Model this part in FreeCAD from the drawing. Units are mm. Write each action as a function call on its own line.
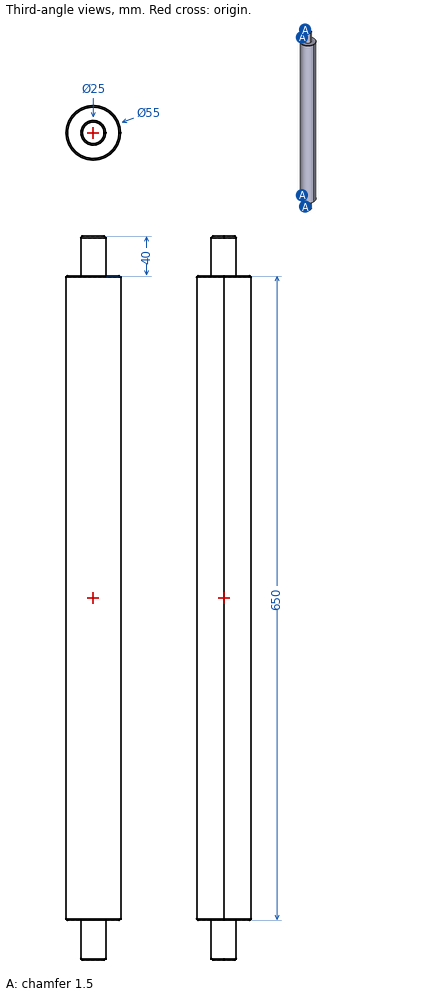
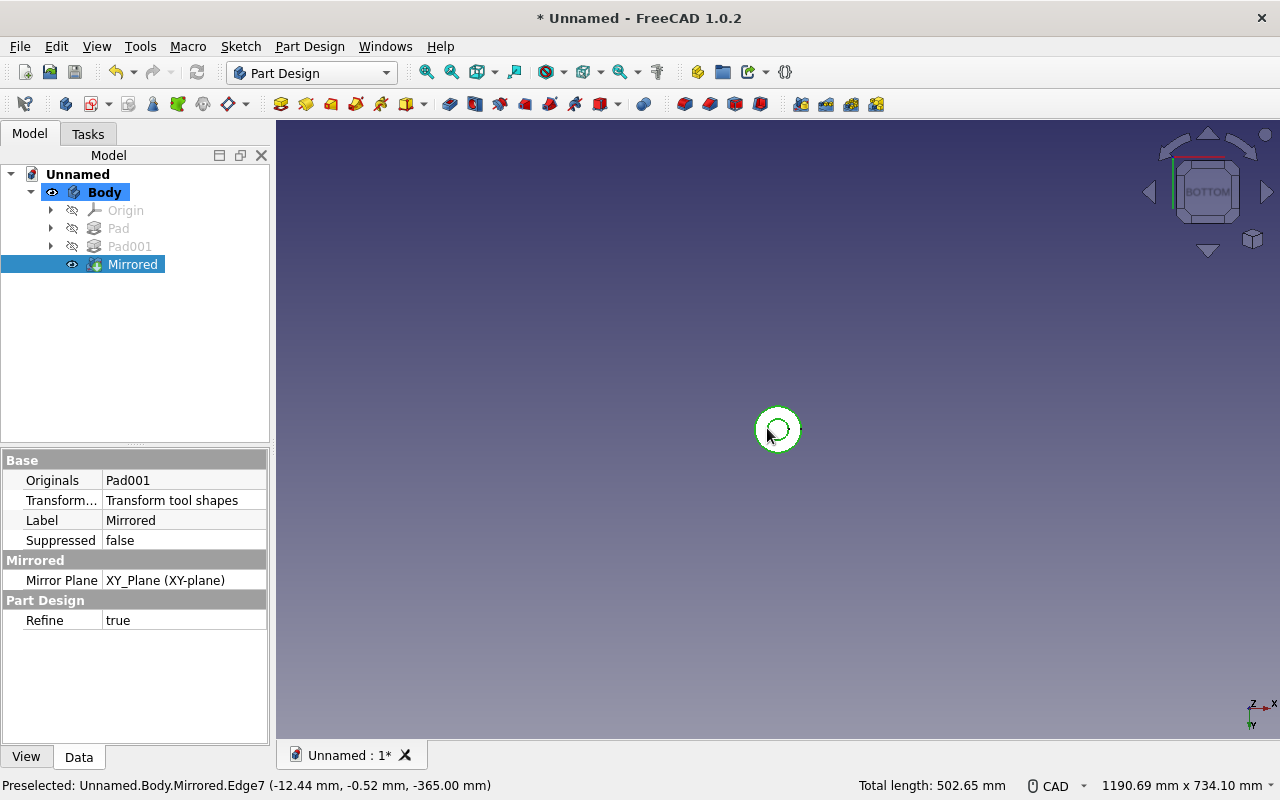
click(710, 104)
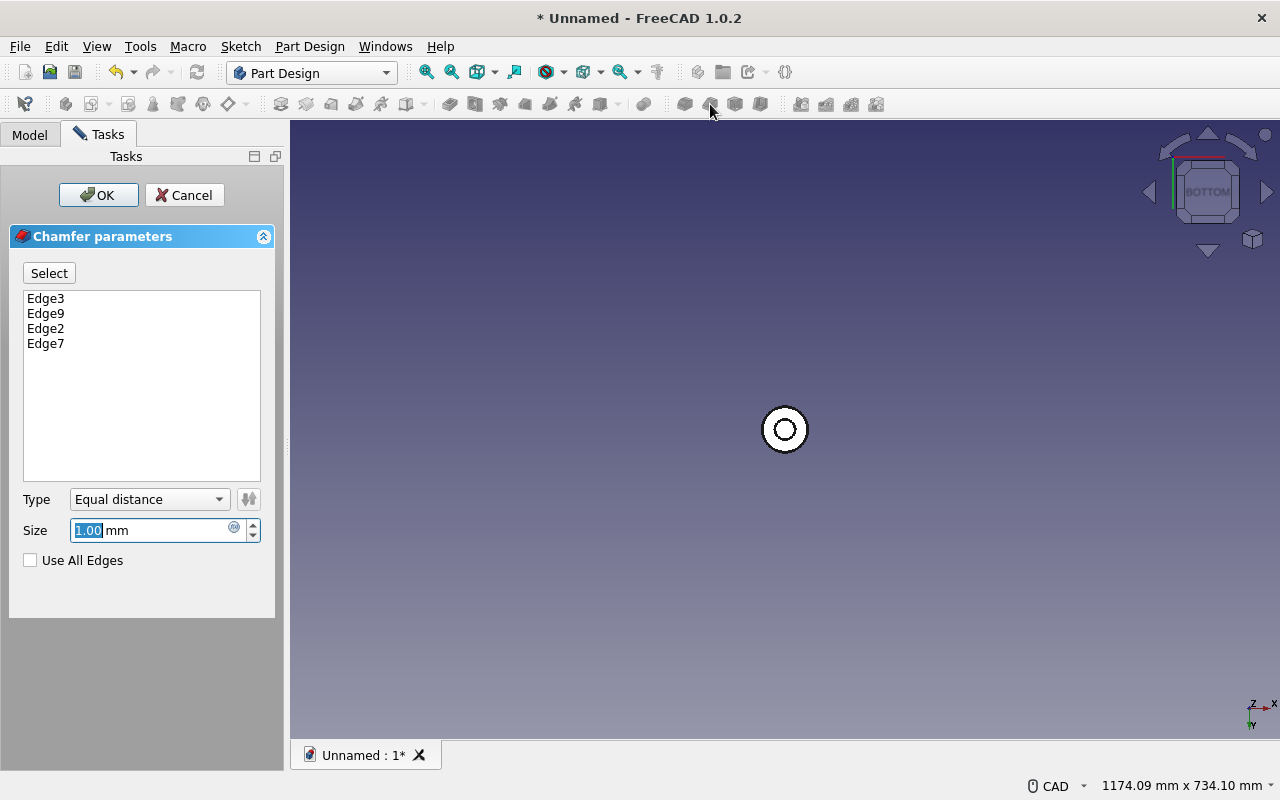
text(1.5)
key(Tab)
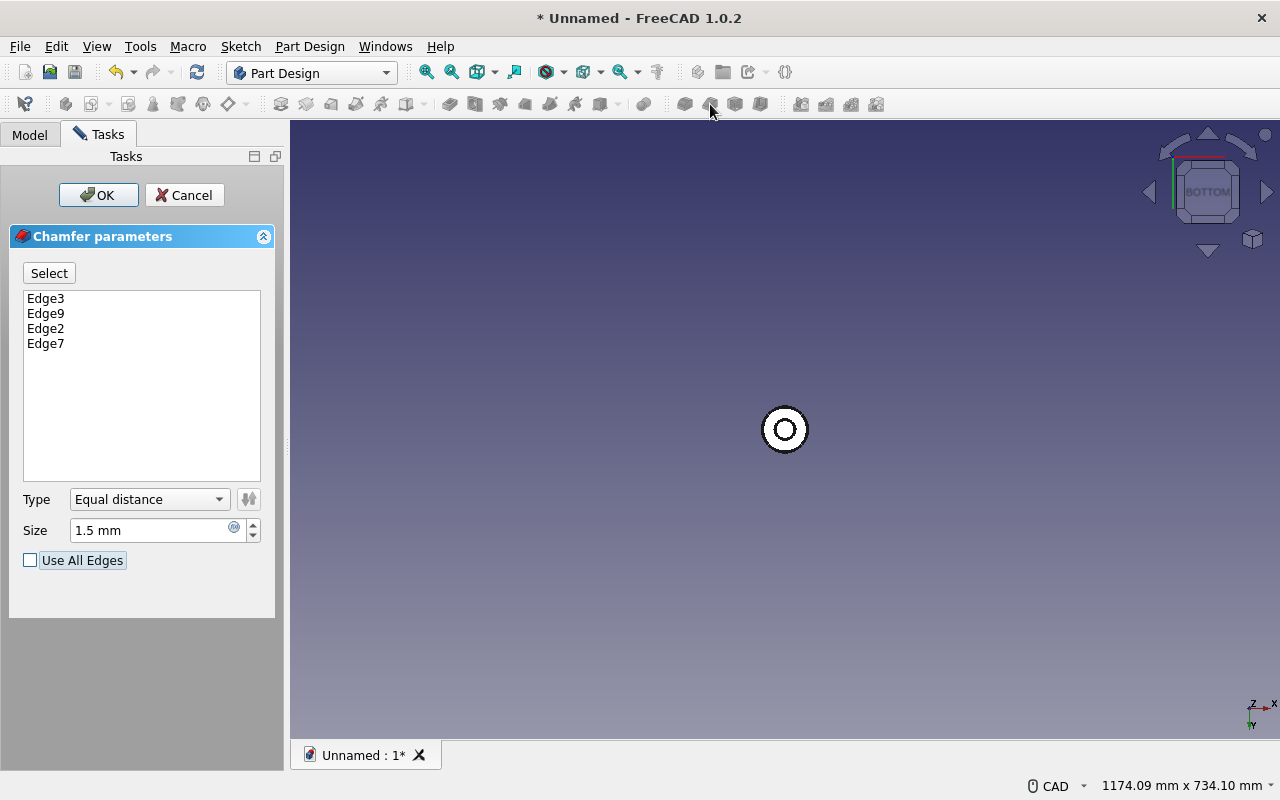
click(99, 195)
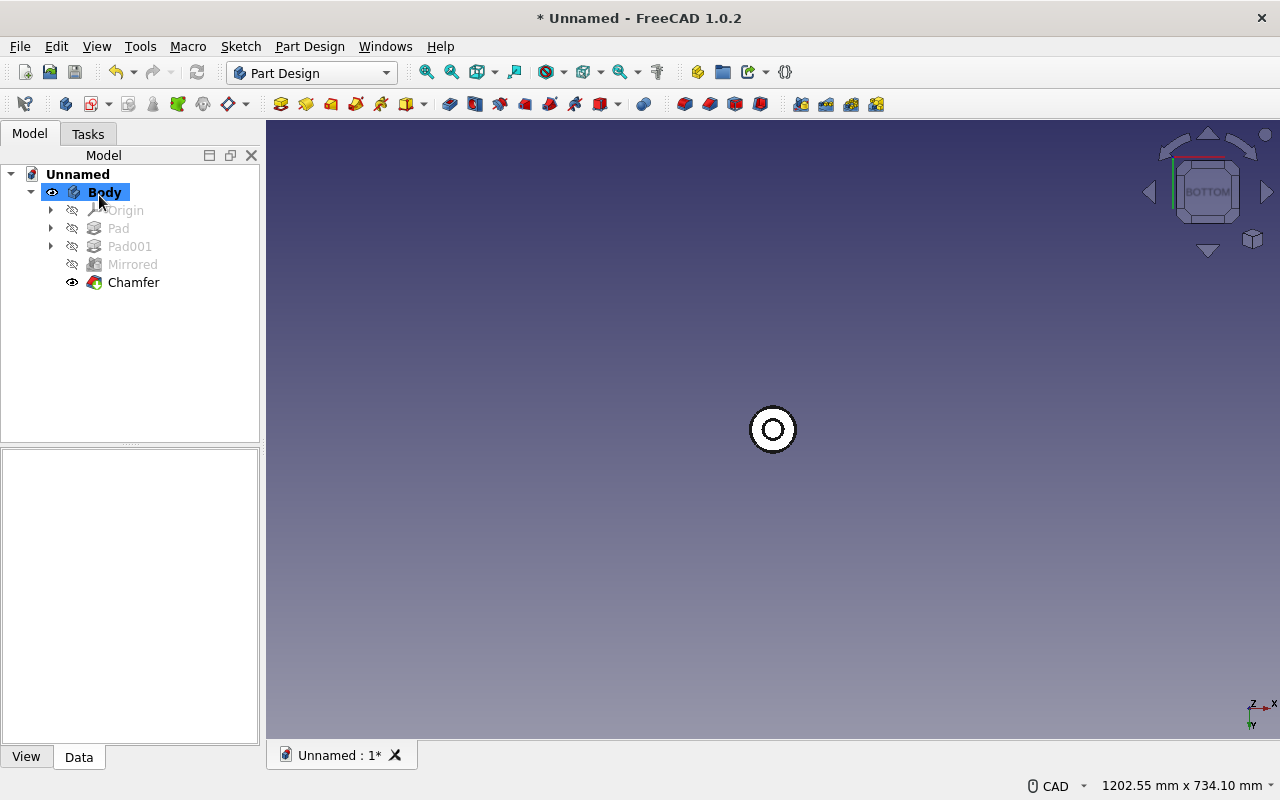
key(0)